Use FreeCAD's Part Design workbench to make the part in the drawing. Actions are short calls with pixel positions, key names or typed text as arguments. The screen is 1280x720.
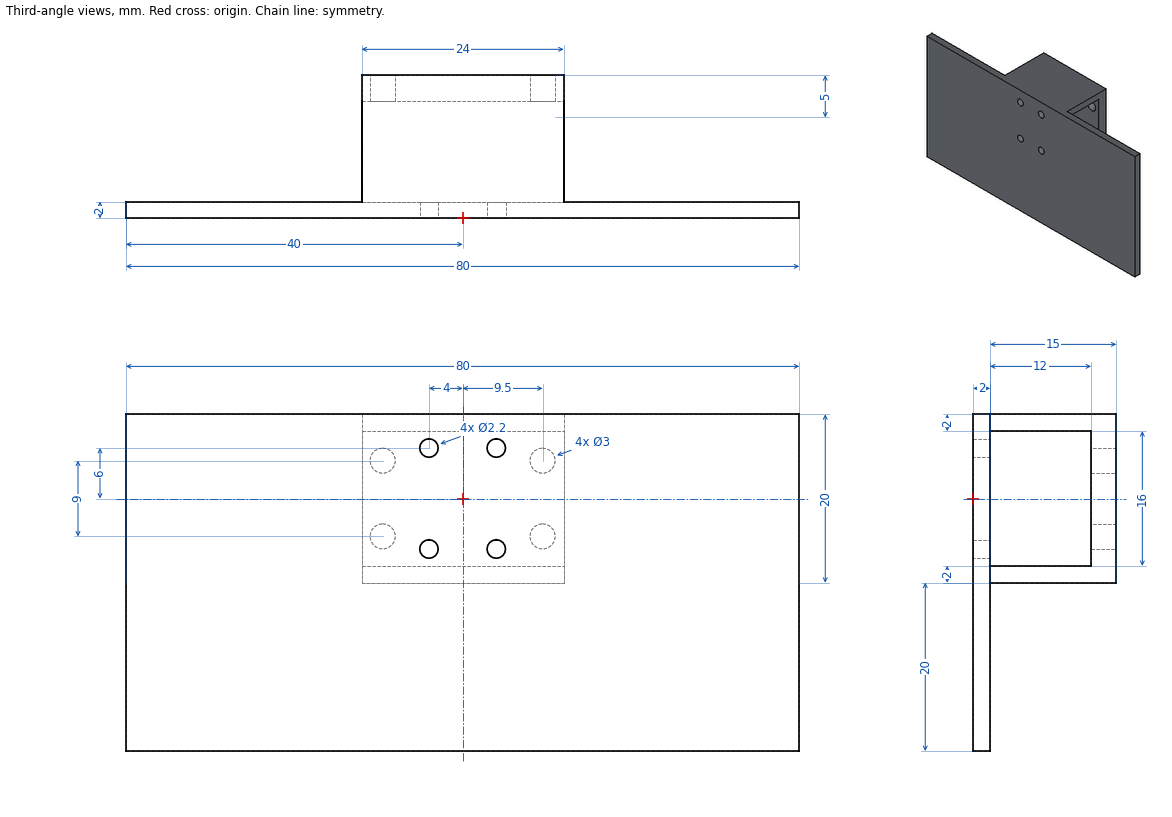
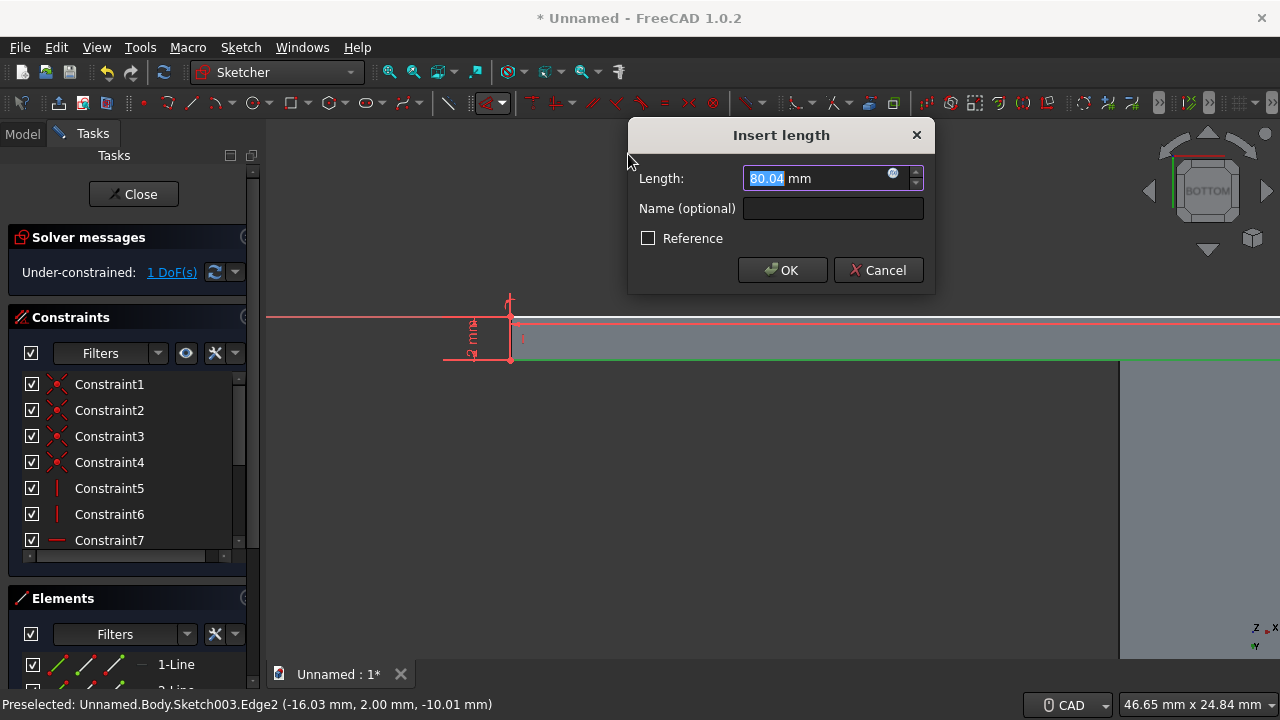
text(80)
key(Return)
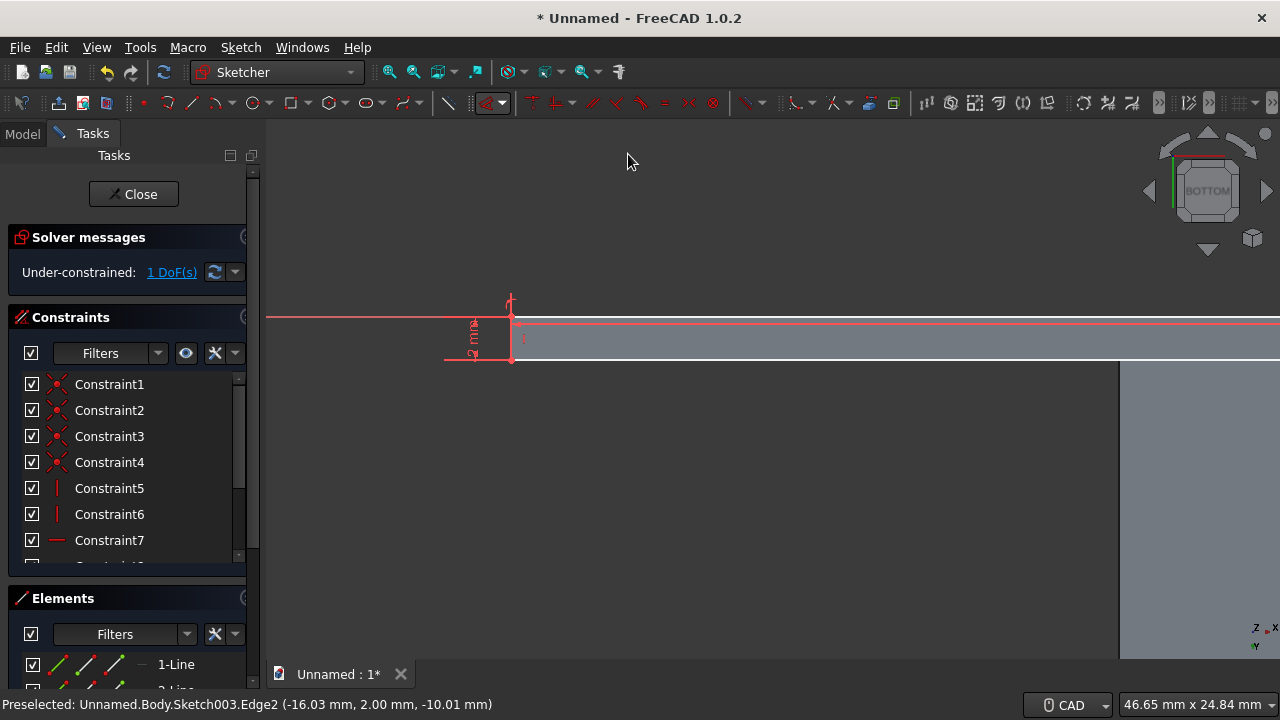
click(511, 317)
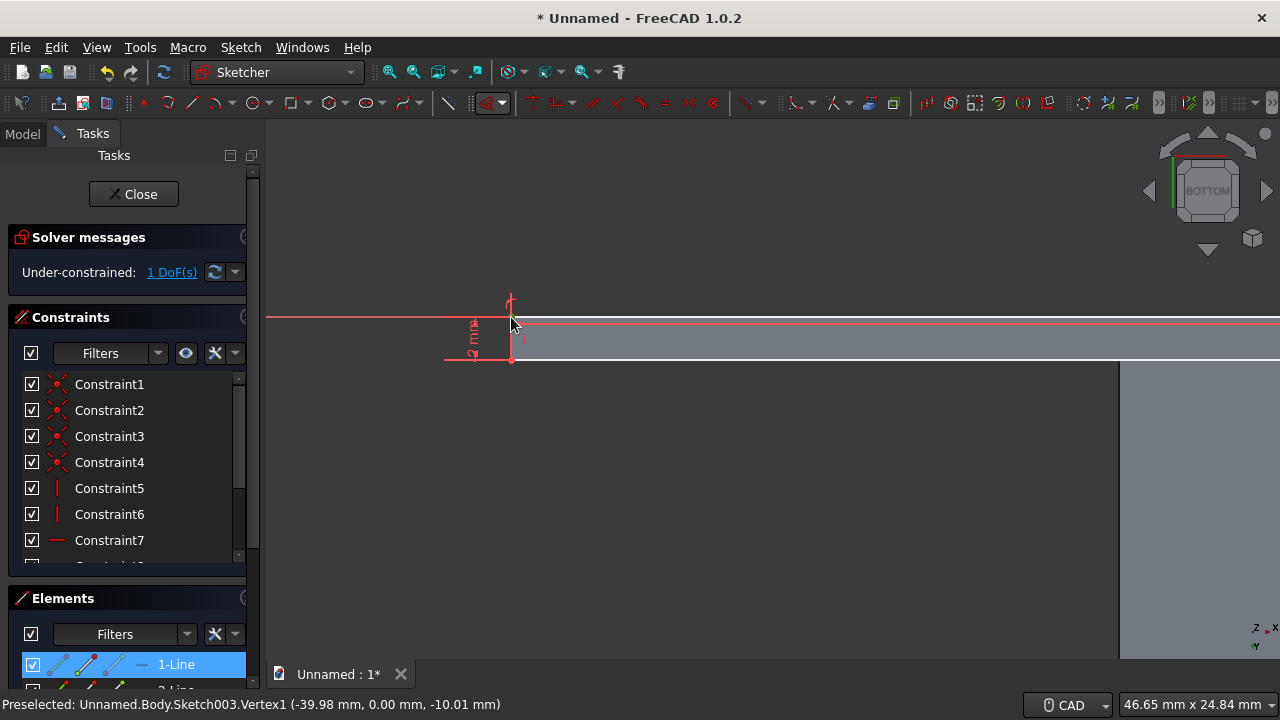
key(l)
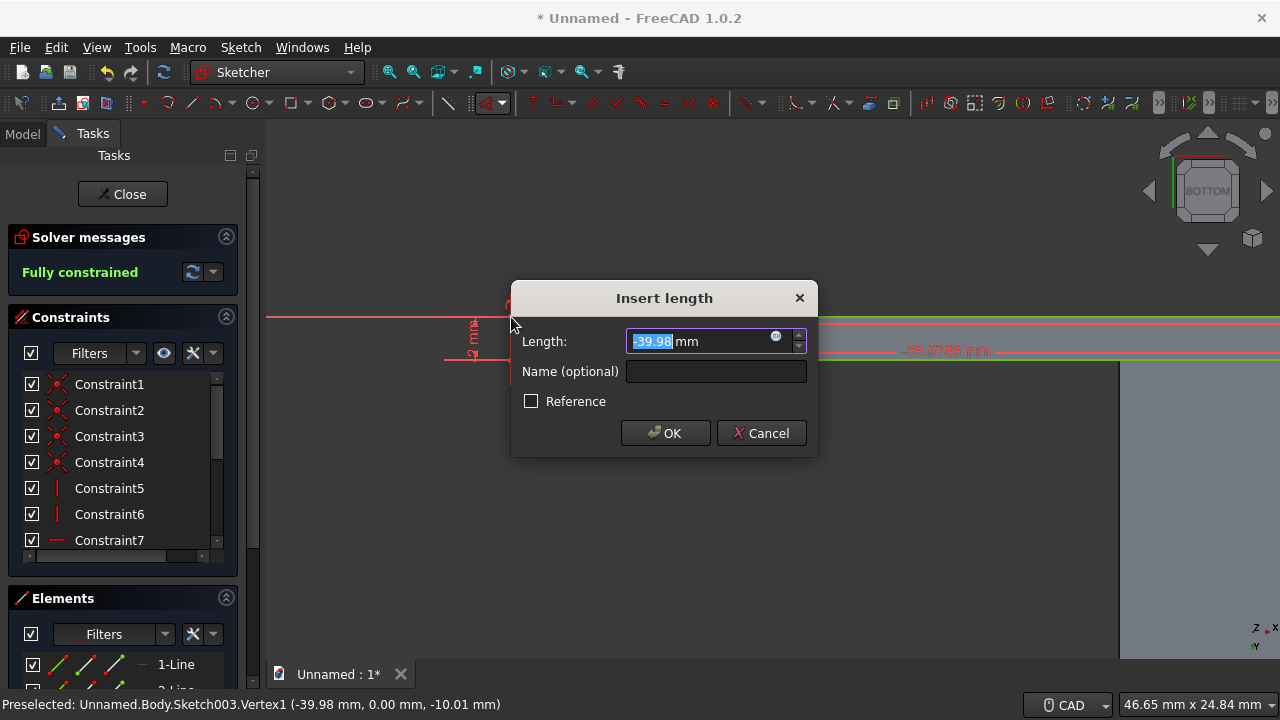
text(-40)
key(Return)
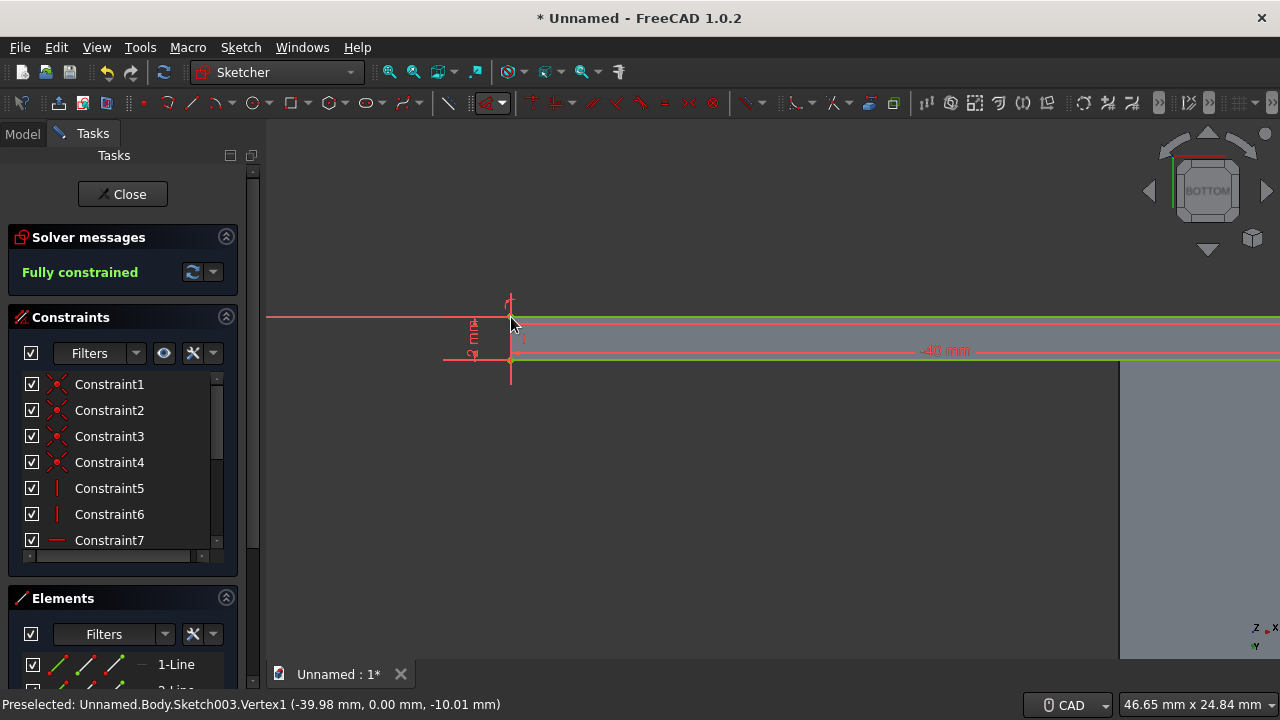
click(123, 194)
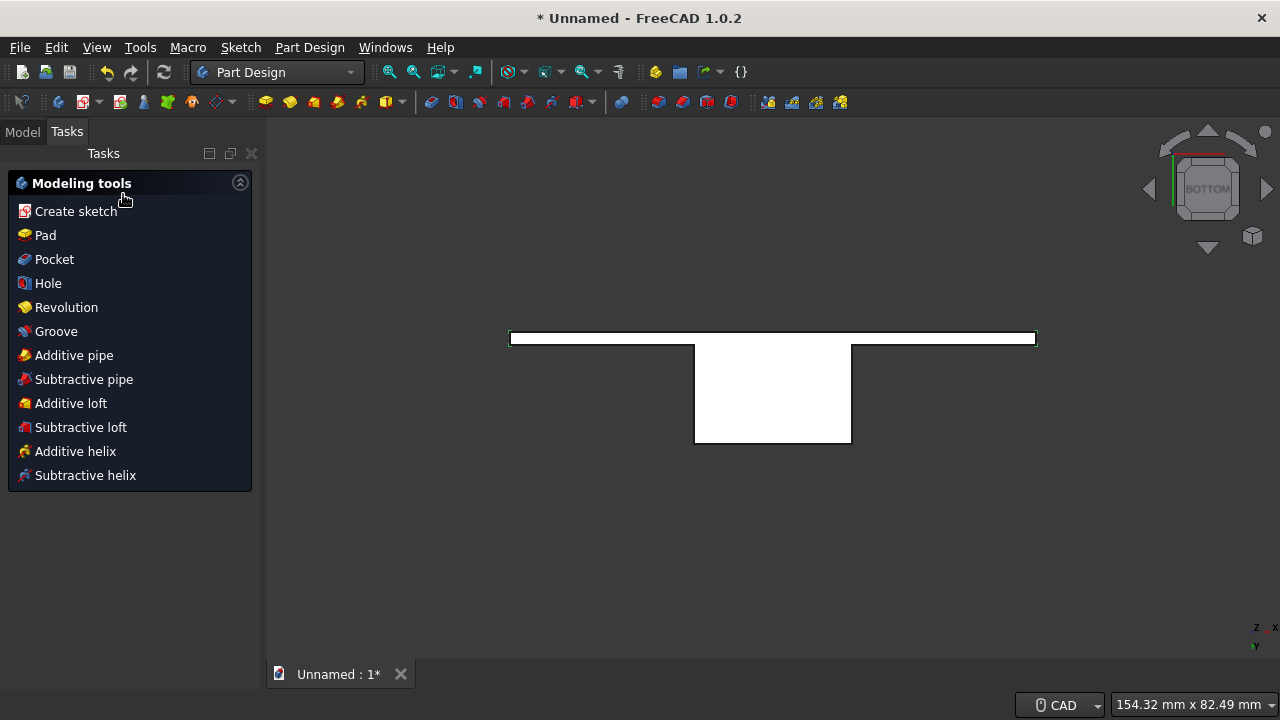
click(266, 102)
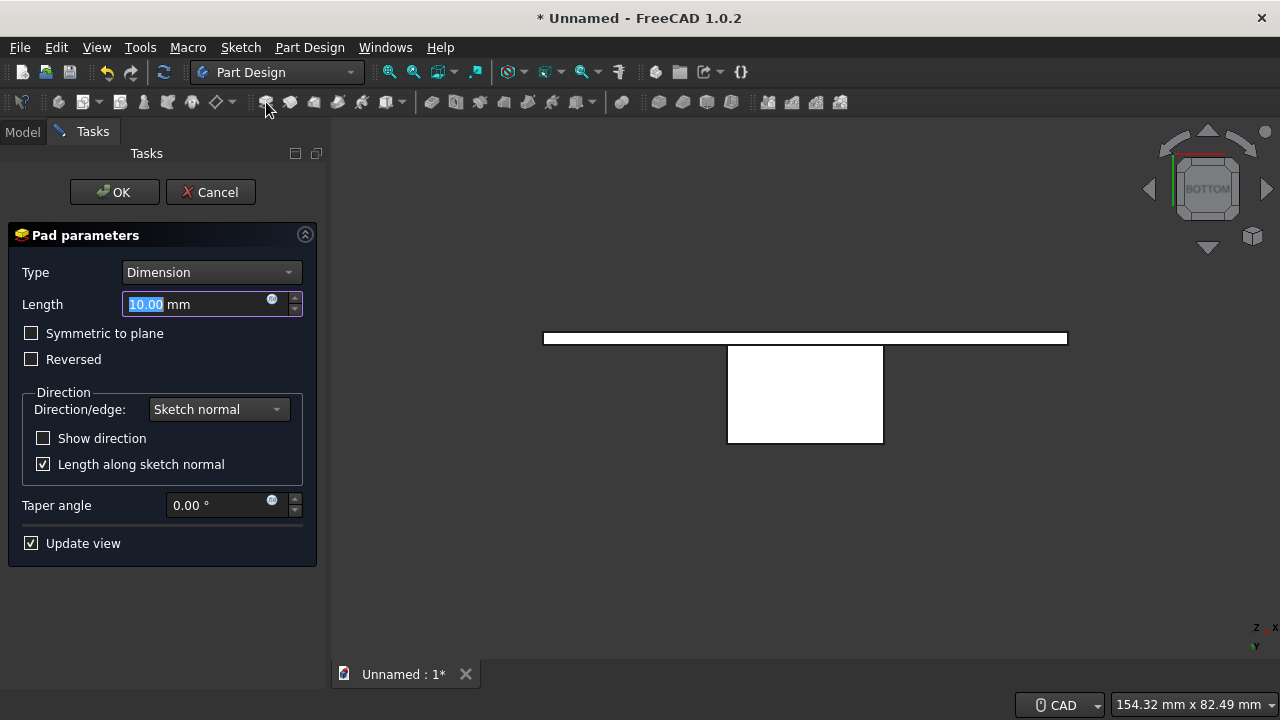
text(20)
key(Tab)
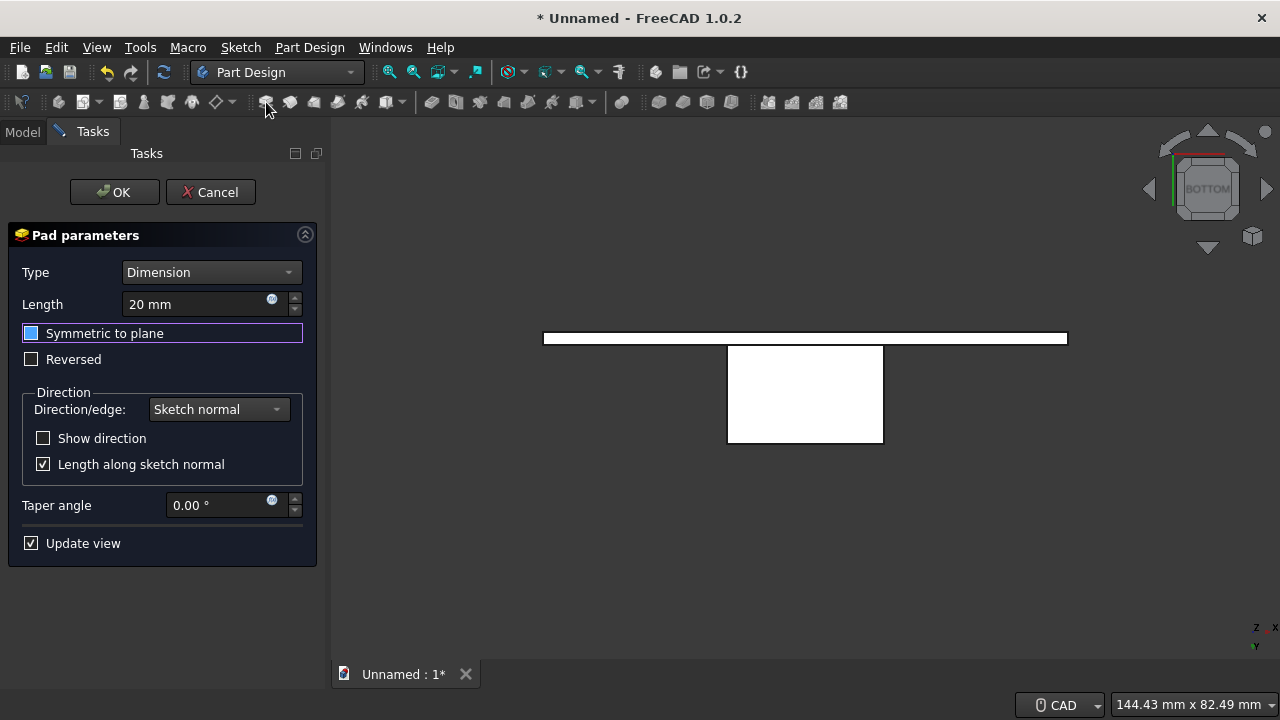
click(115, 192)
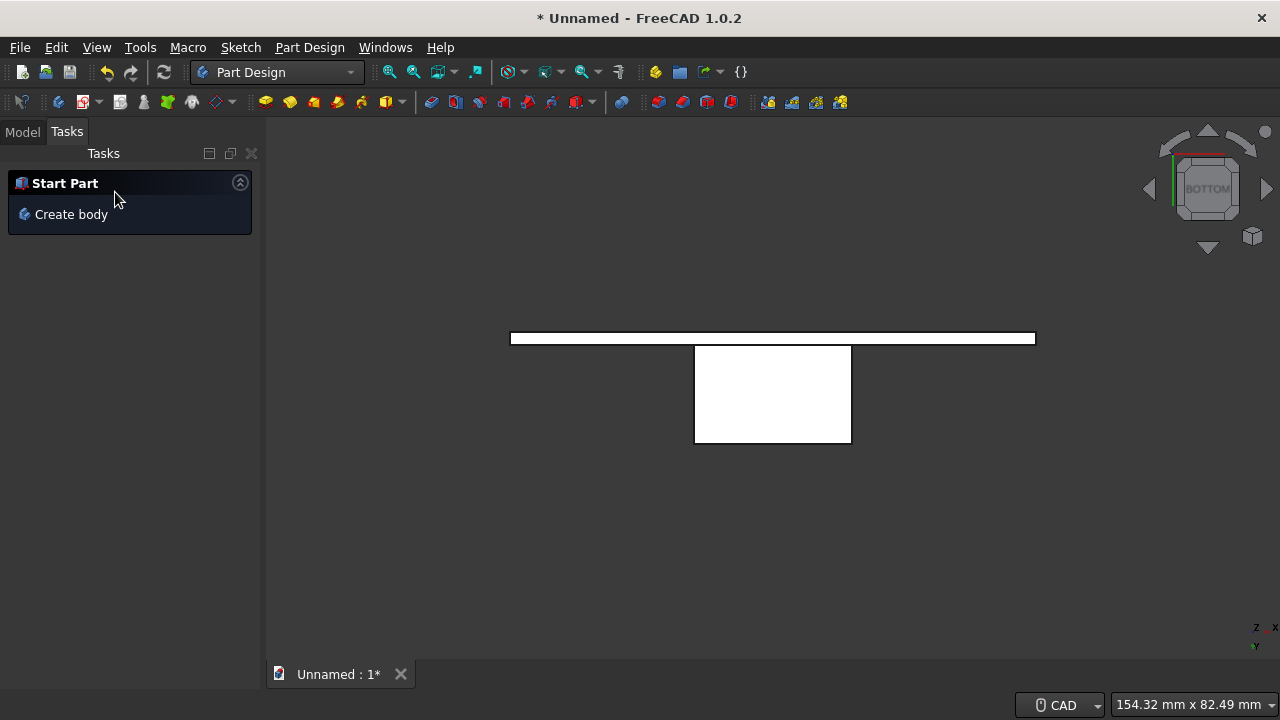
key(0)